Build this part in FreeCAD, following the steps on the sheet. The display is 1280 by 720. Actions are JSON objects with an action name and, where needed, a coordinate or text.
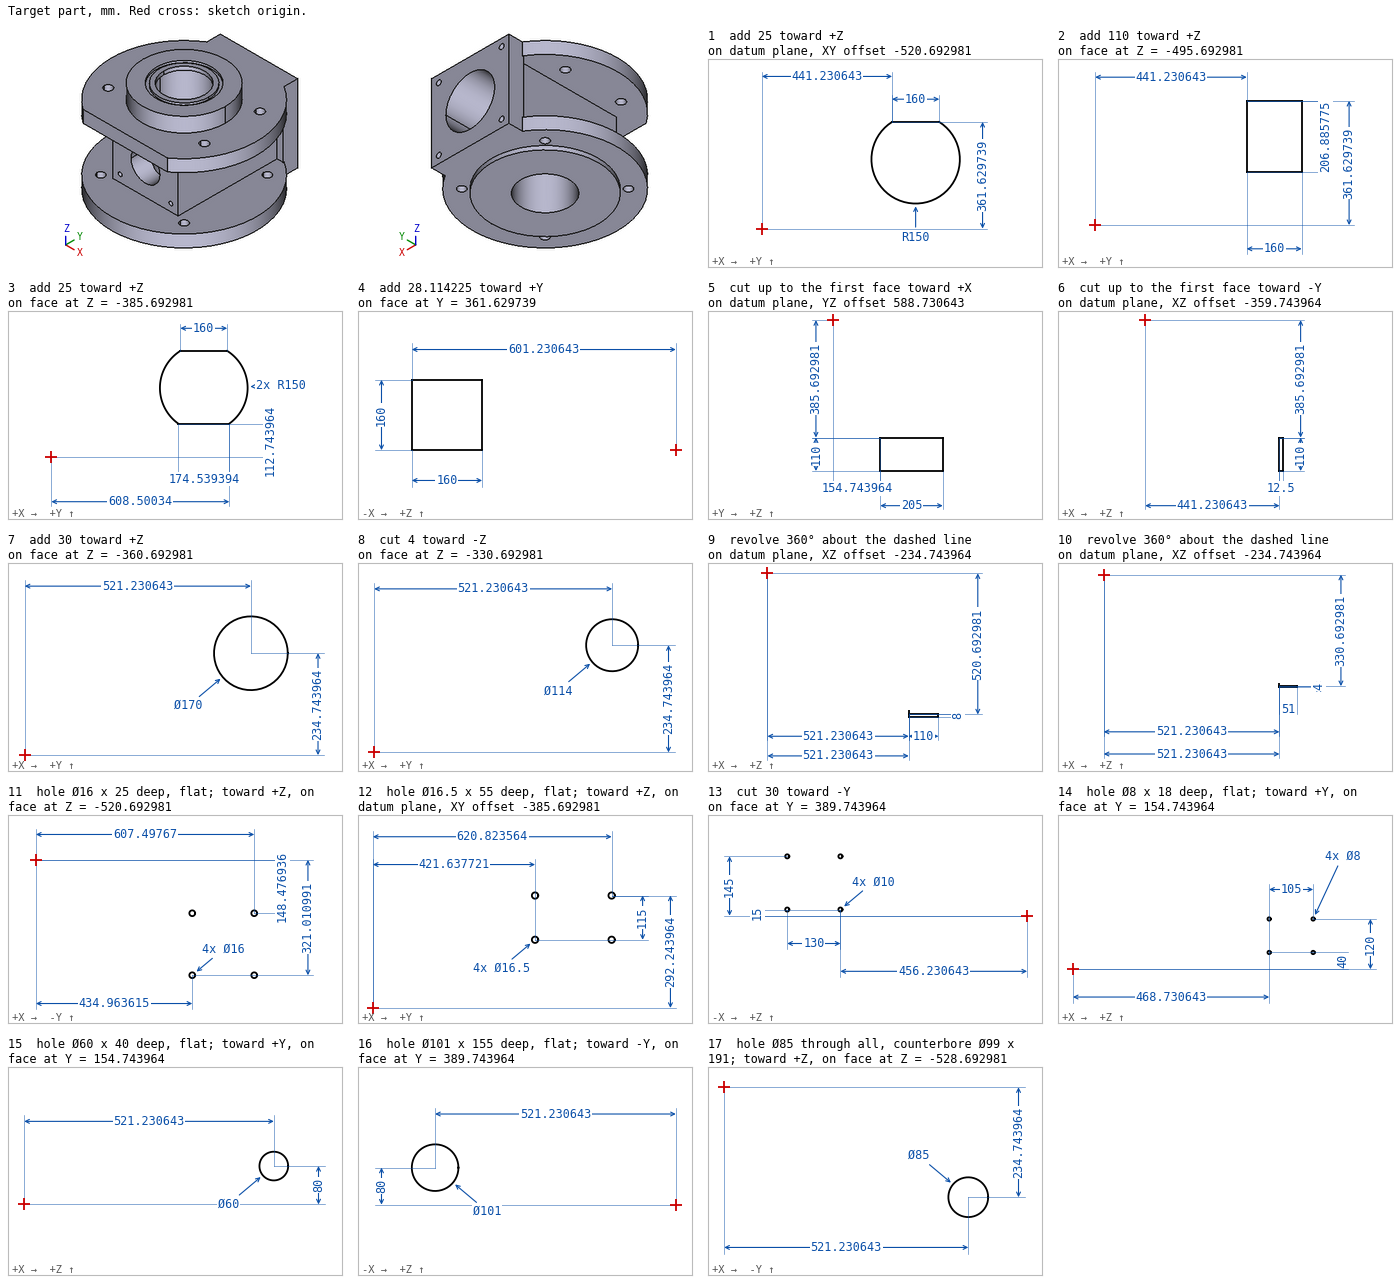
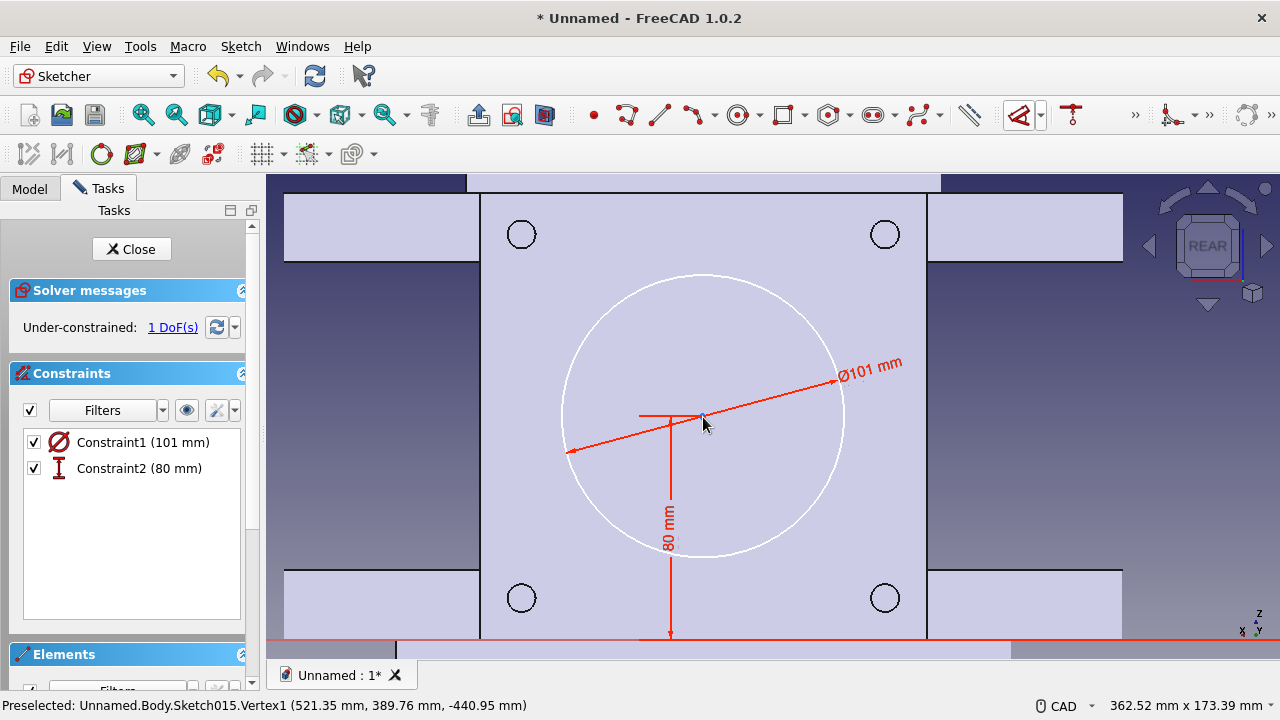
{"action": "left_click", "coordinate": [703, 416]}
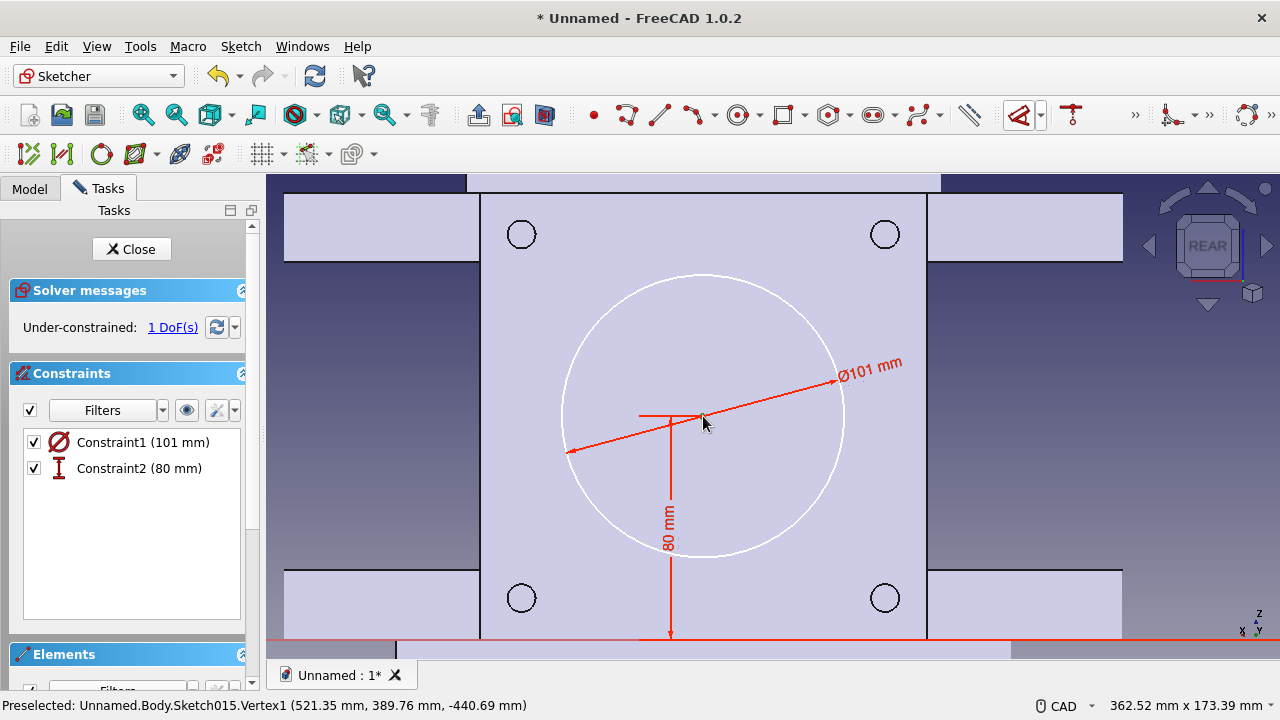
{"action": "left_click", "coordinate": [1040, 116]}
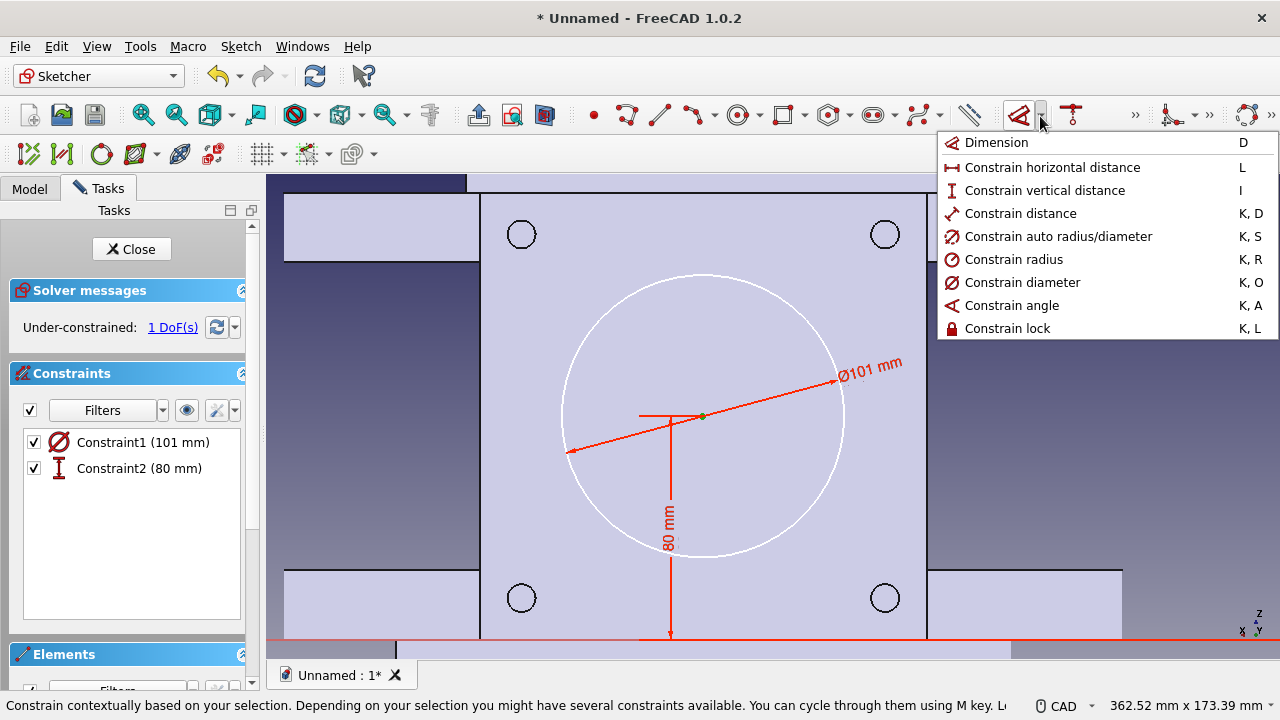
{"action": "left_click", "coordinate": [1108, 168]}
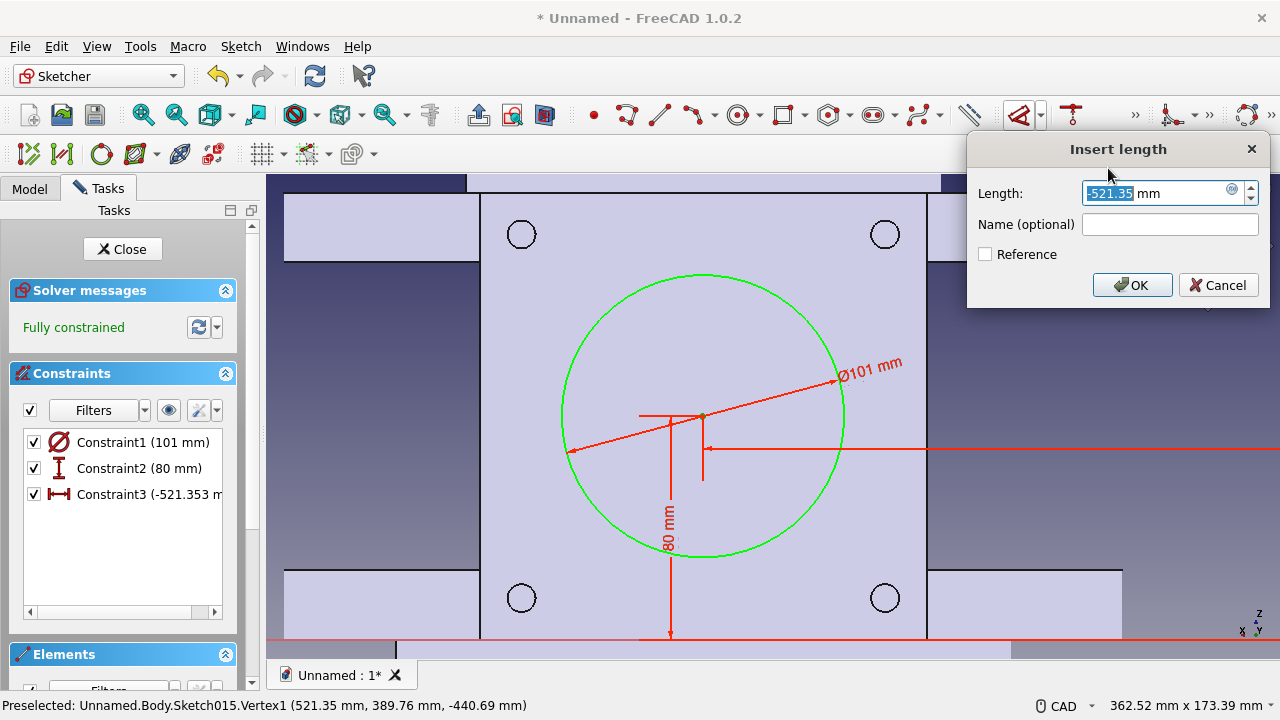
{"action": "type", "text": "-521.230643"}
{"action": "key", "text": "Return"}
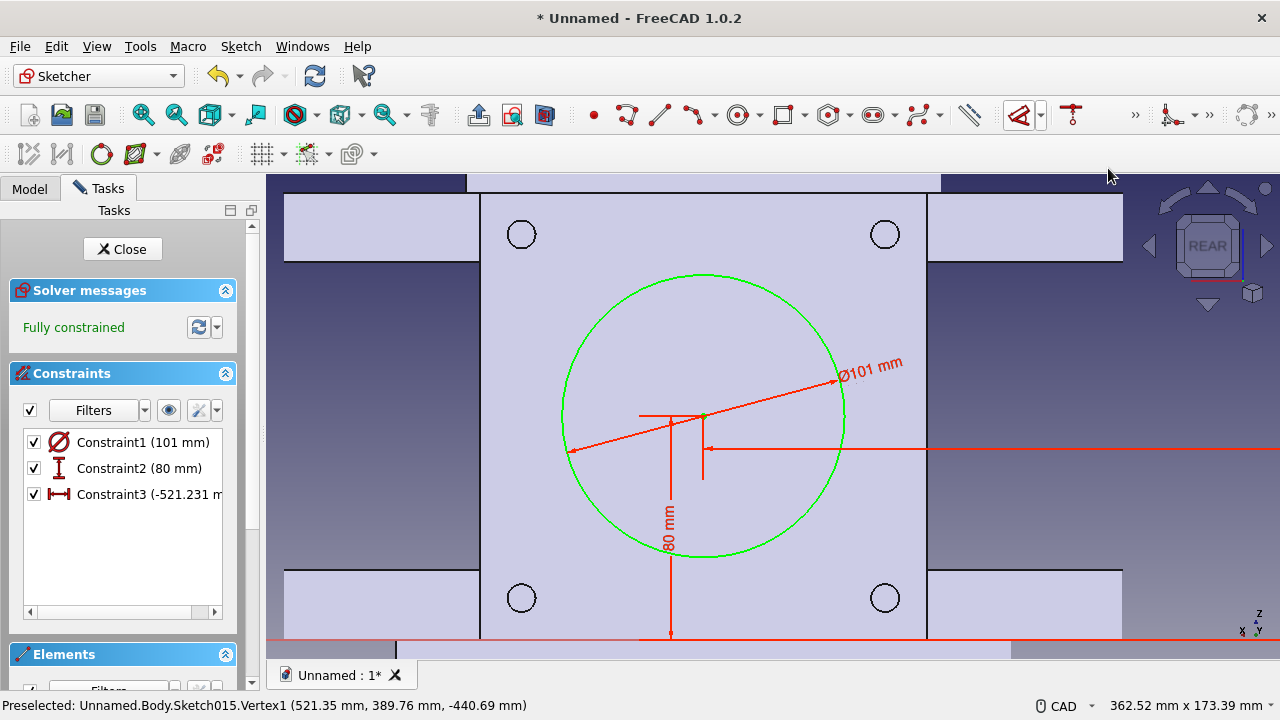
{"action": "left_click", "coordinate": [123, 249]}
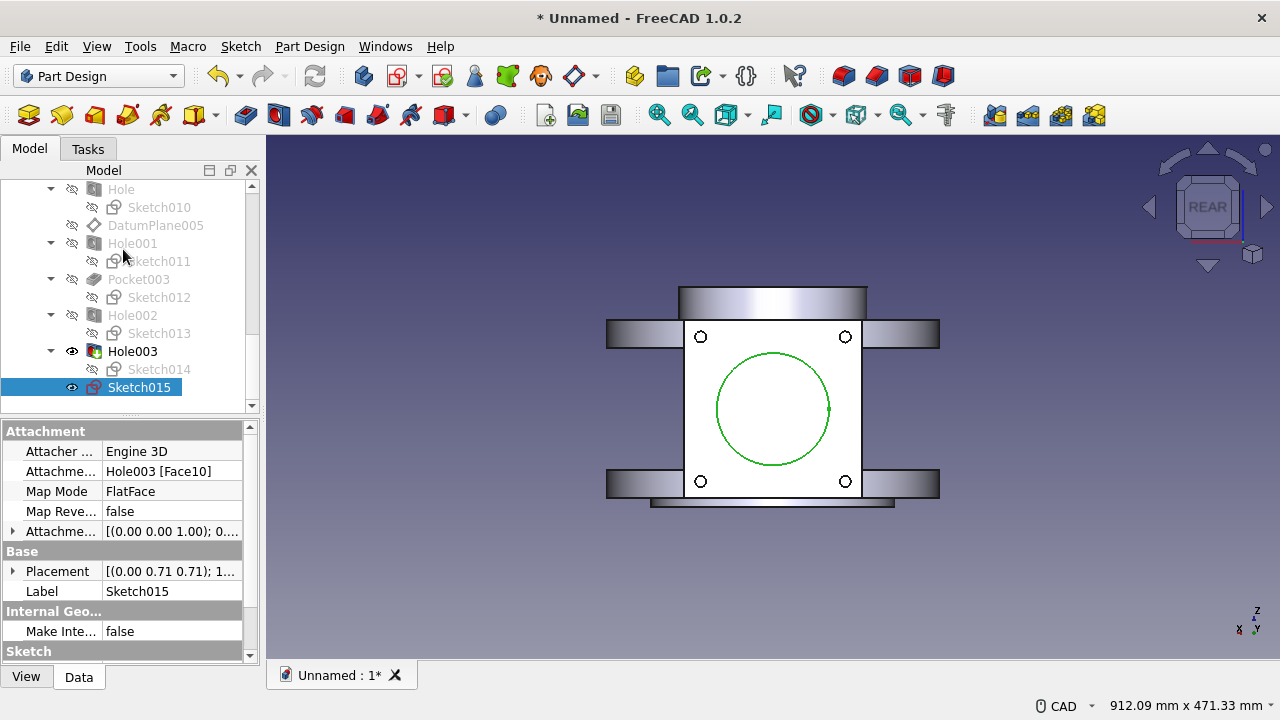
{"action": "left_click", "coordinate": [279, 116]}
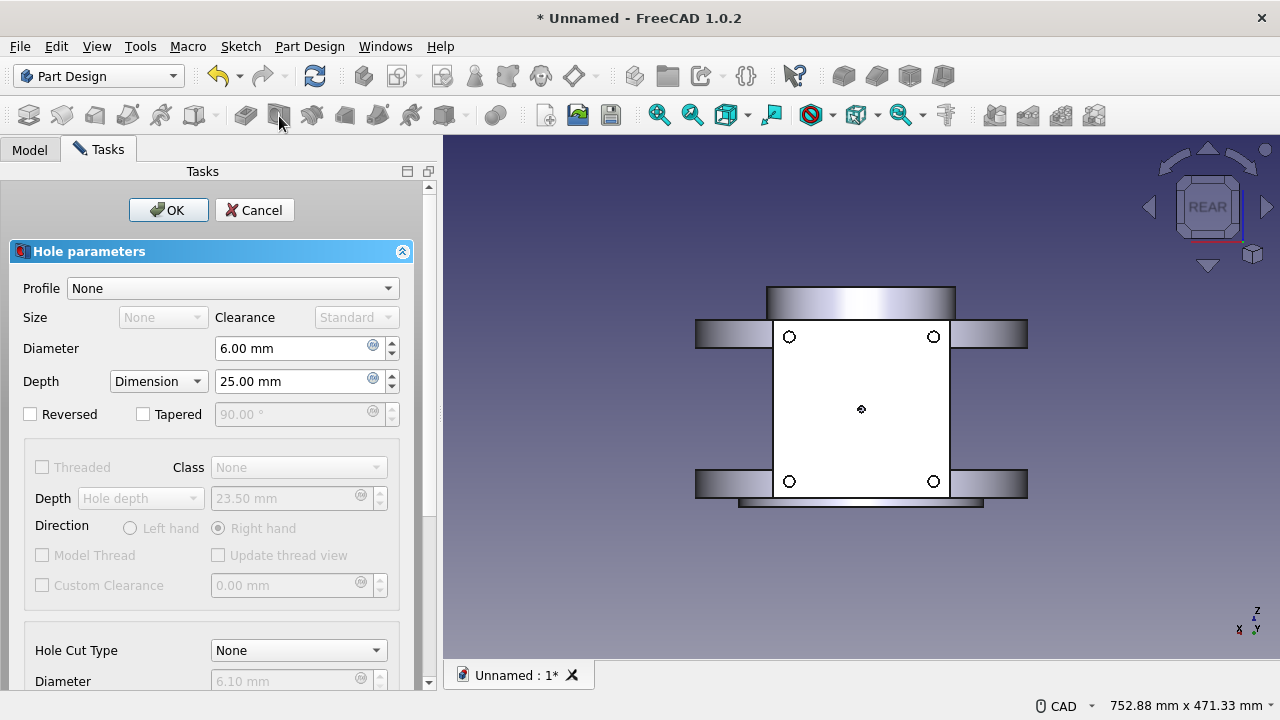
{"action": "triple_click", "coordinate": [300, 348]}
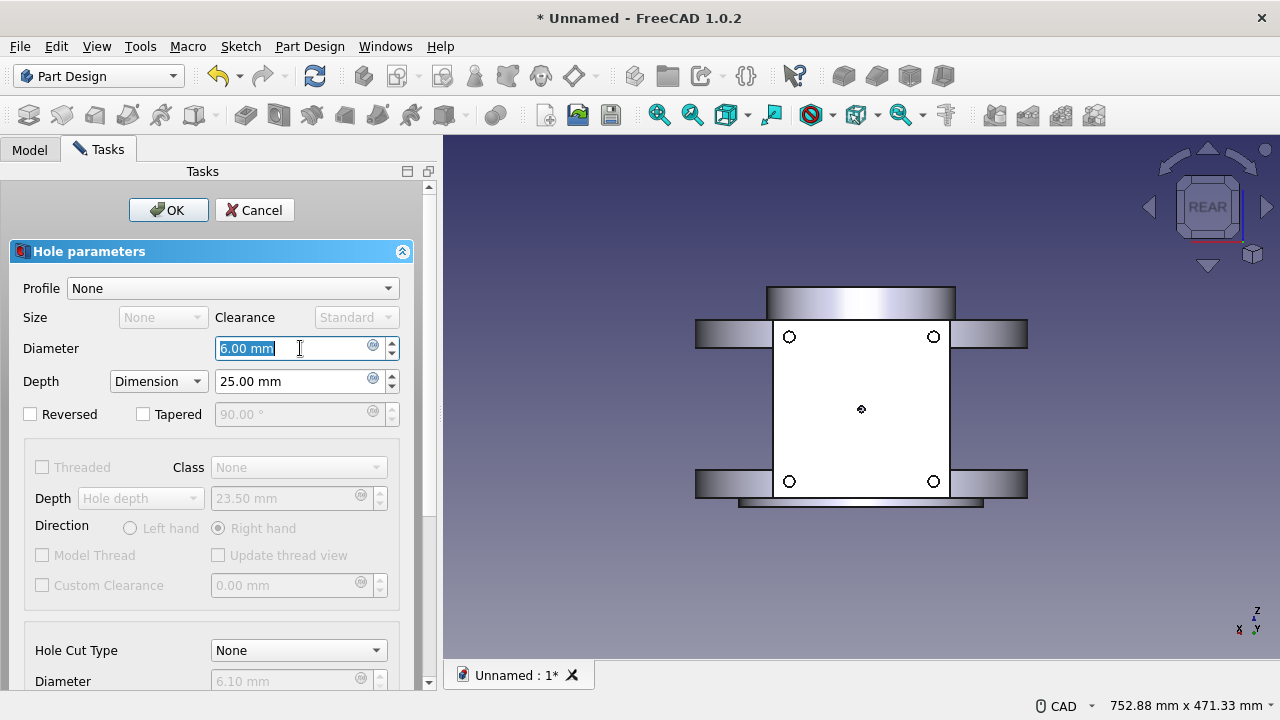
{"action": "type", "text": "101"}
{"action": "key", "text": "Tab"}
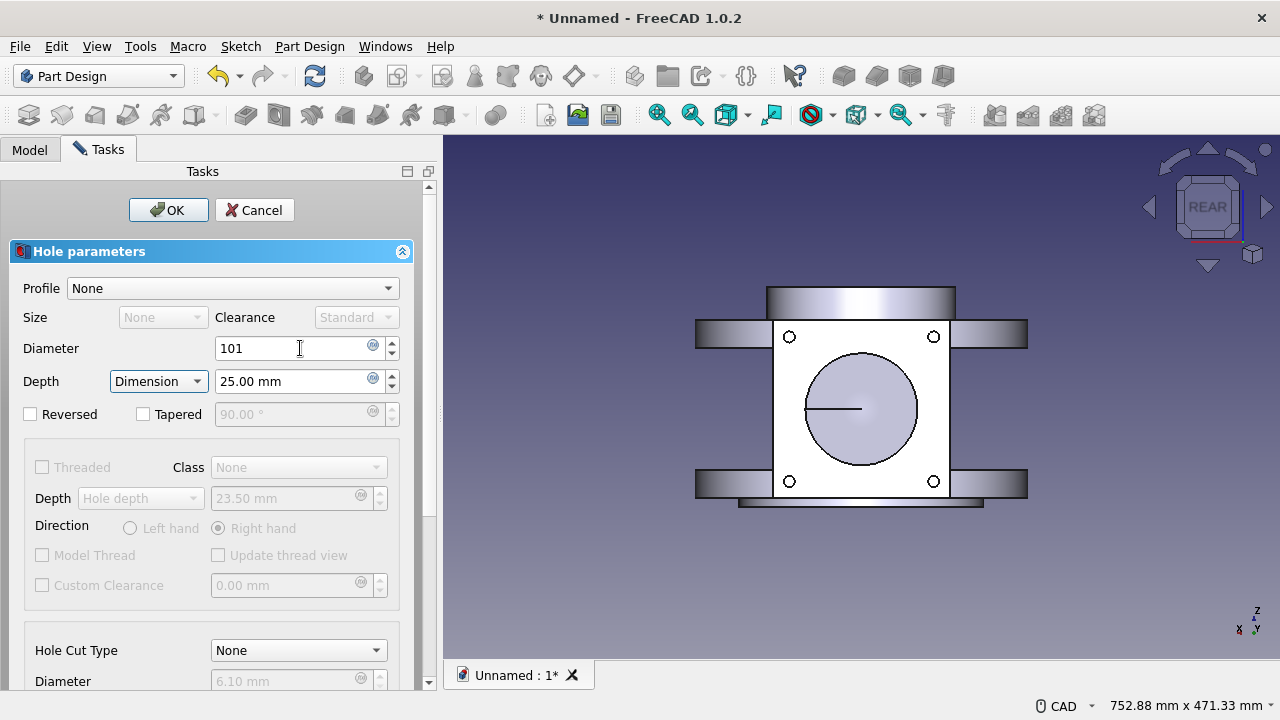
{"action": "triple_click", "coordinate": [300, 382]}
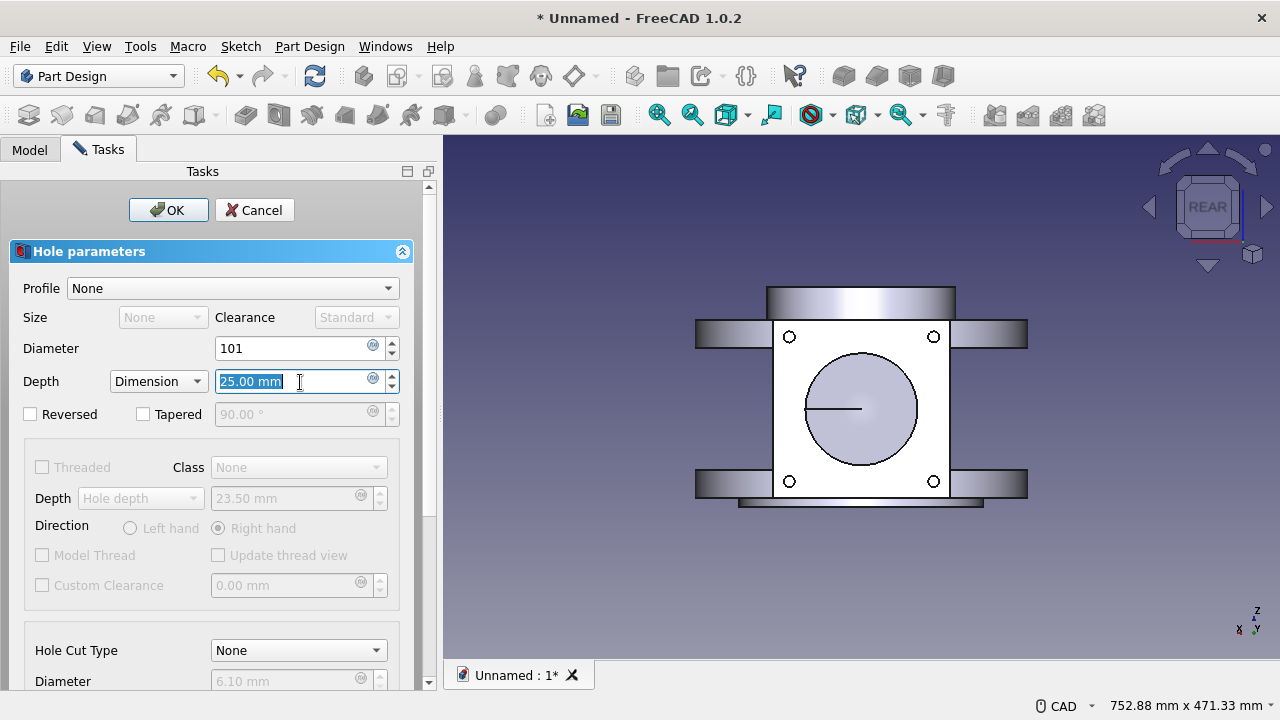
{"action": "type", "text": "155"}
{"action": "key", "text": "Tab"}